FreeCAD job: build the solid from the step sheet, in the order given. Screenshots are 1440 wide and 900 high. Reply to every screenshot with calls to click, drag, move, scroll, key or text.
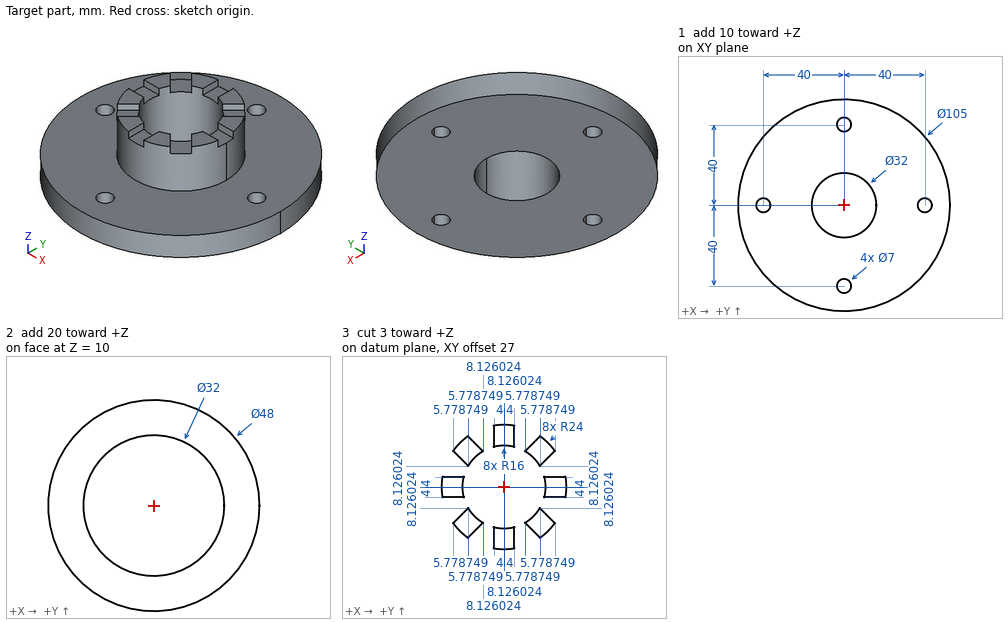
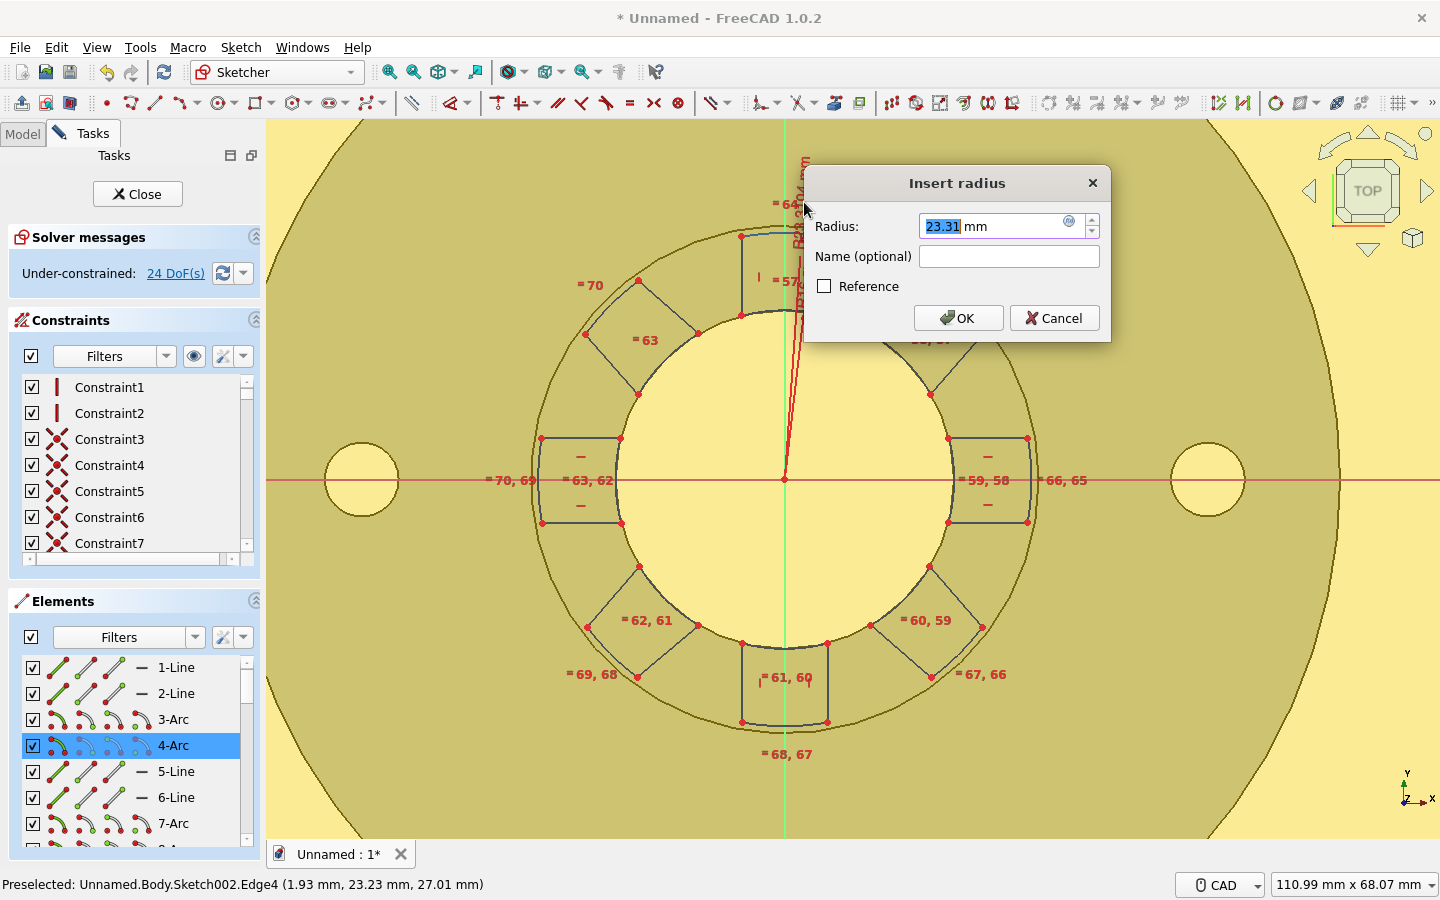
text(24)
key(Return)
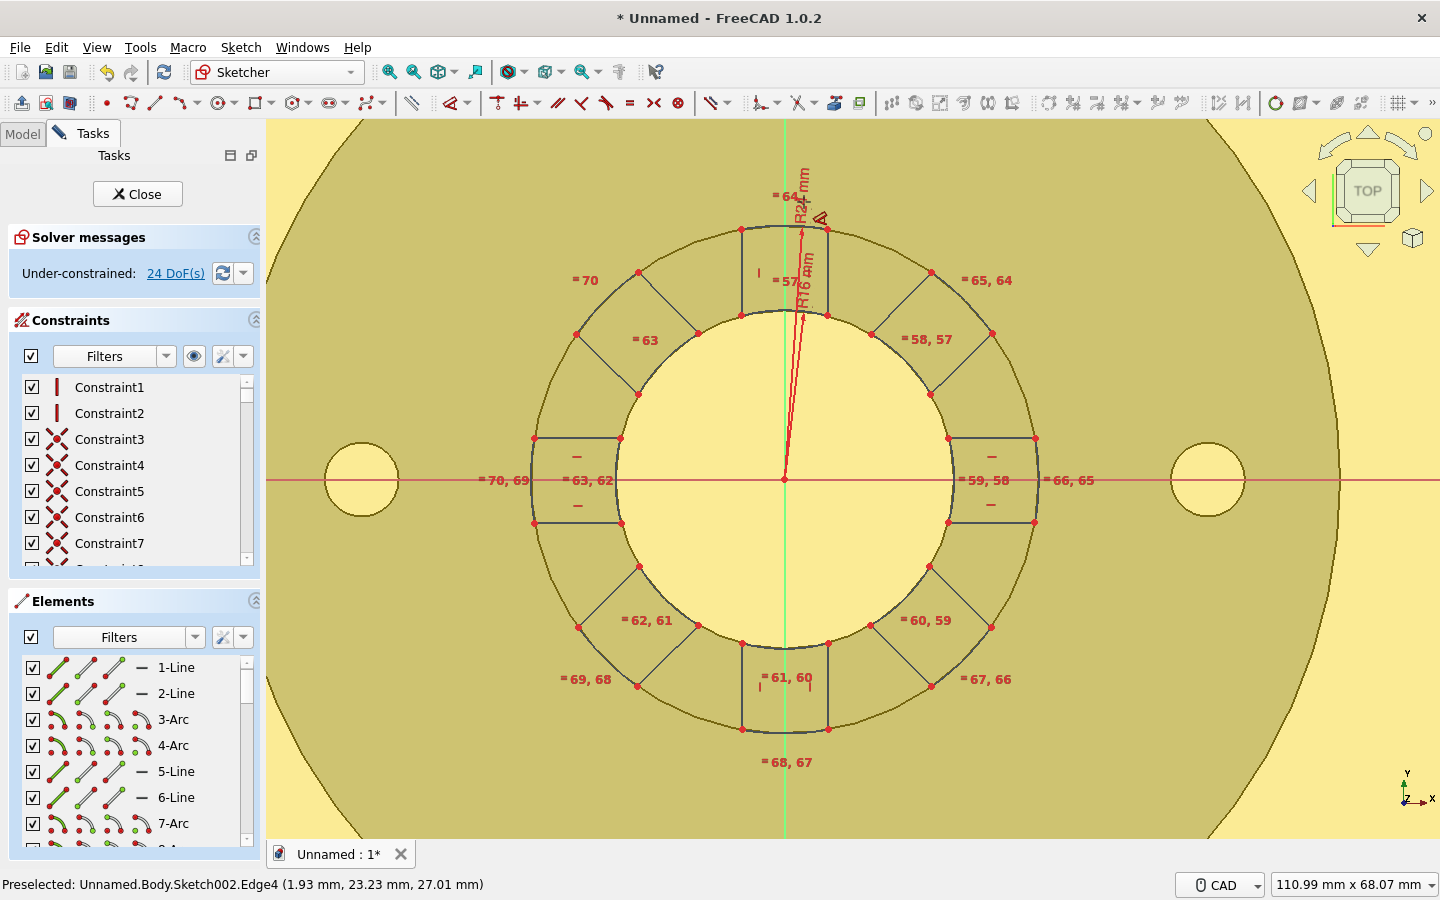
click(742, 229)
click(763, 514)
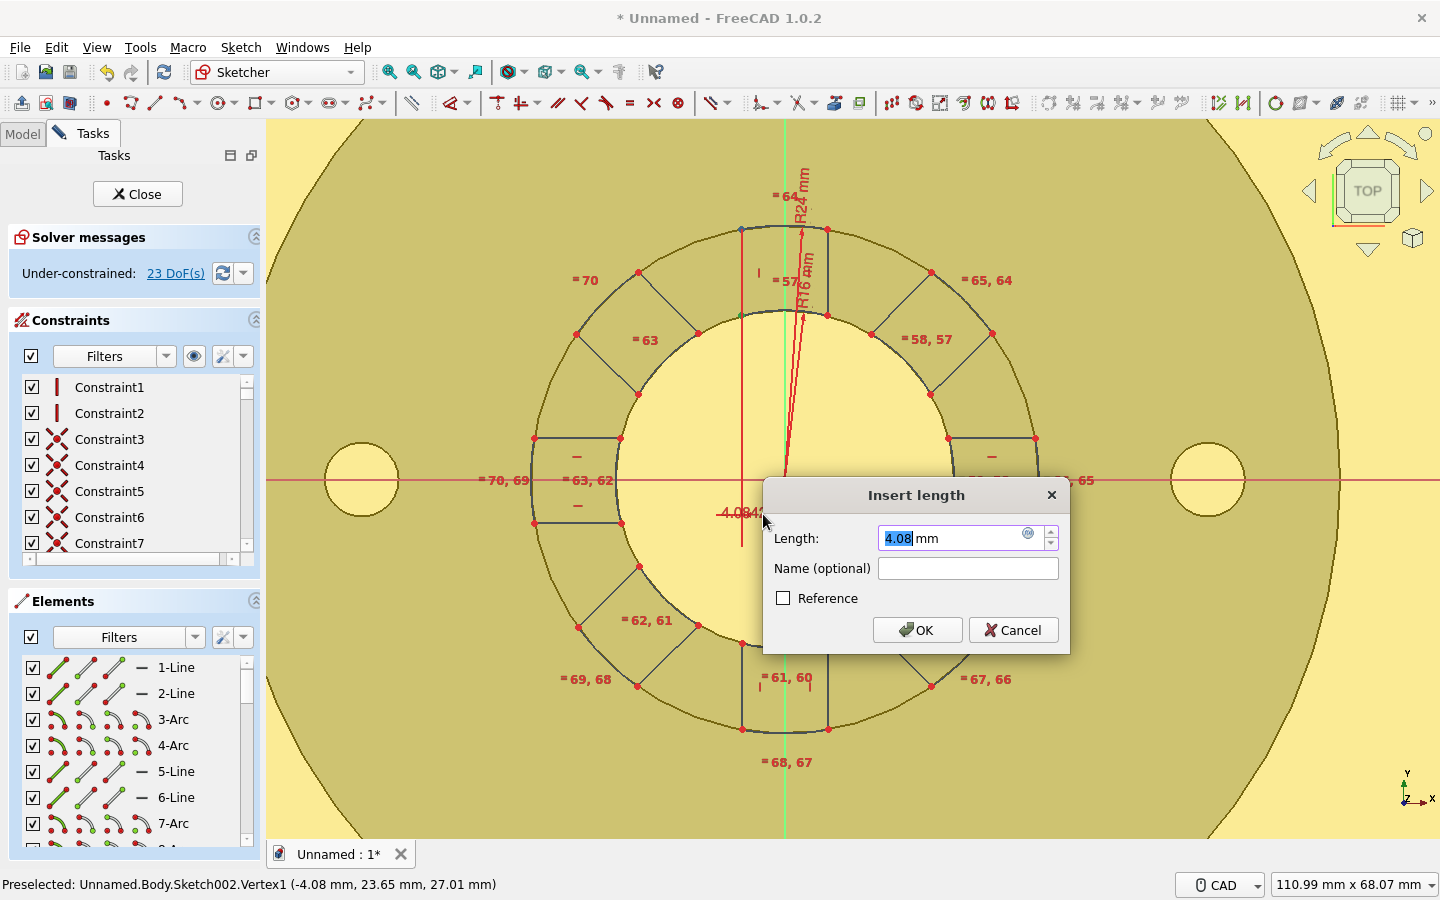
text(4)
key(Return)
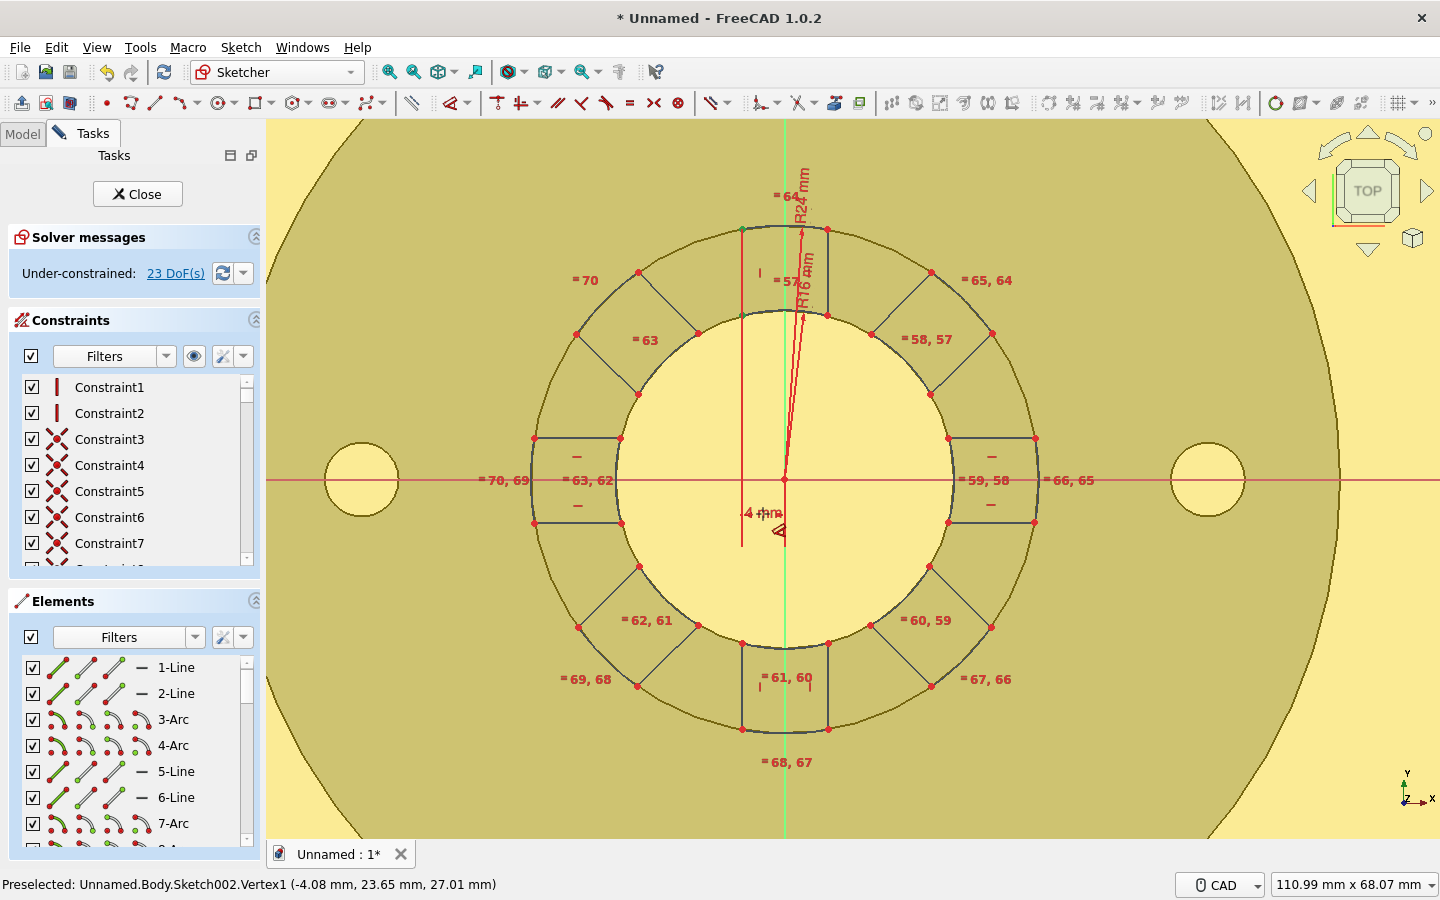
click(828, 316)
click(806, 258)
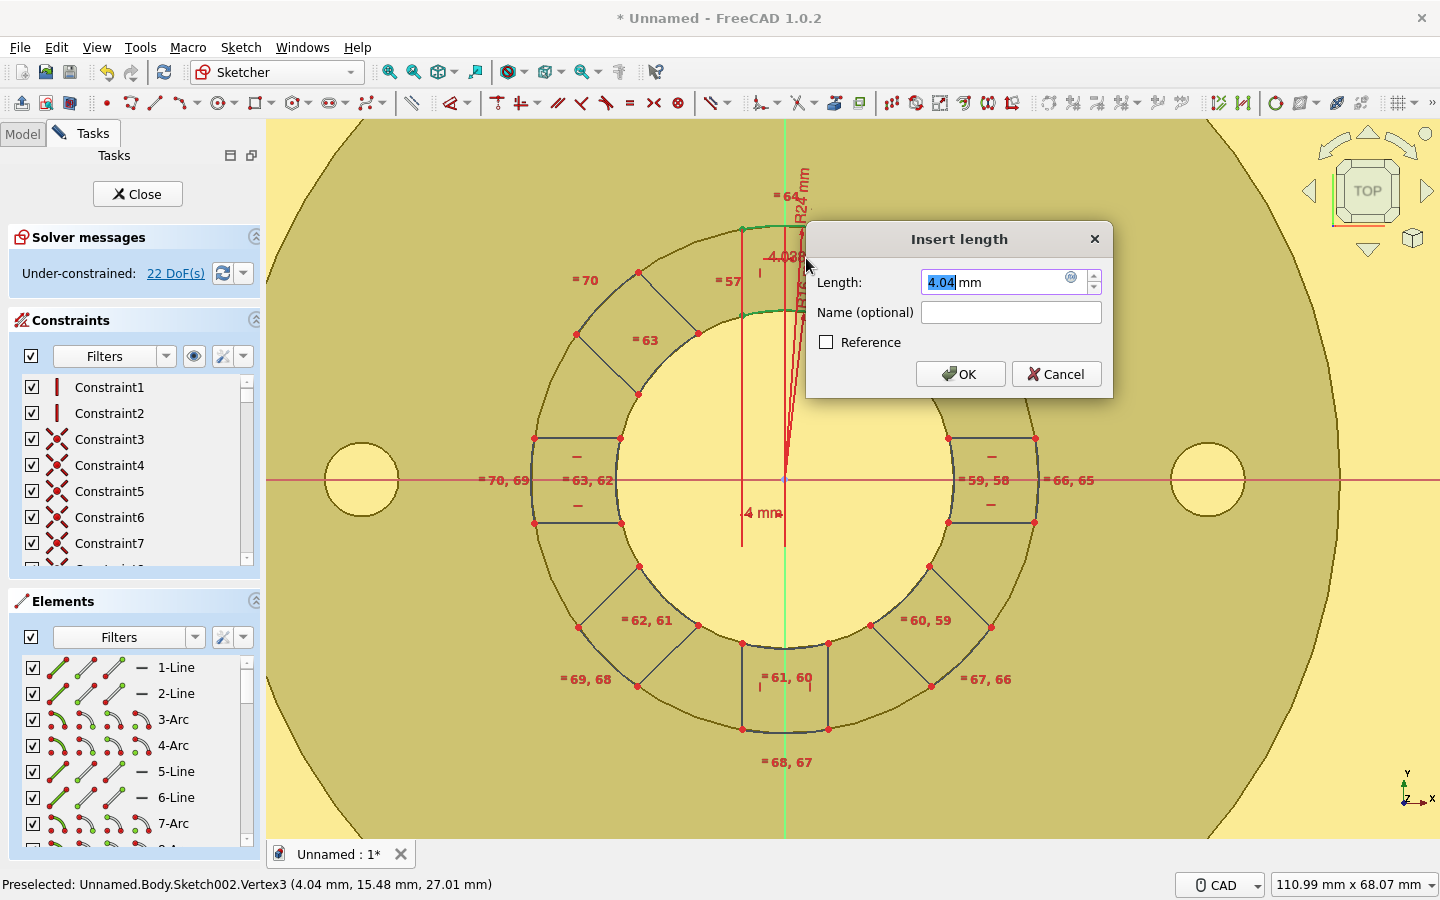
text(4)
key(Return)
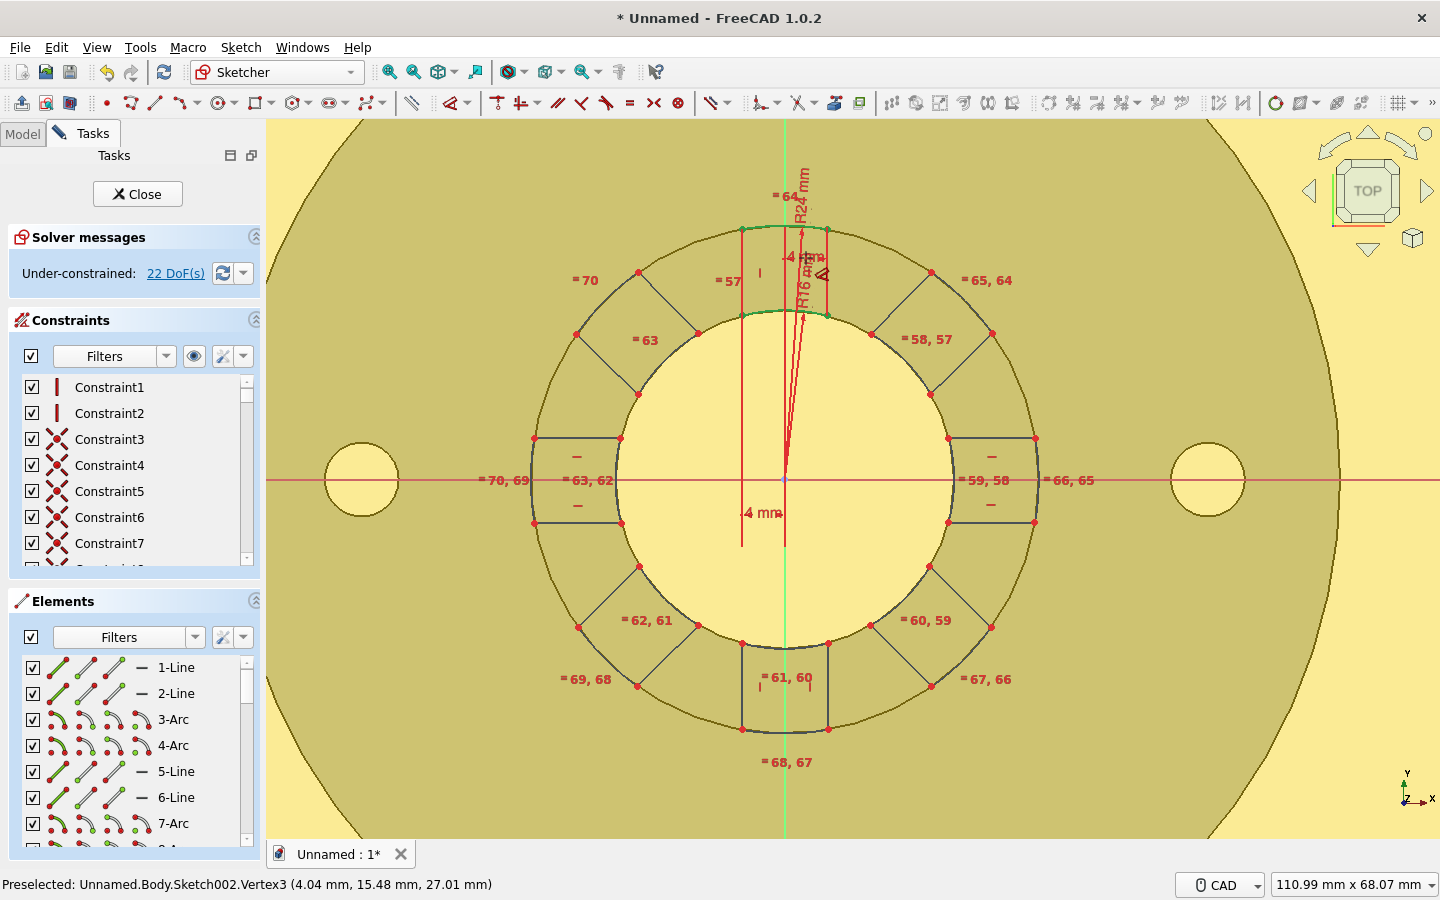
click(1035, 438)
click(1069, 459)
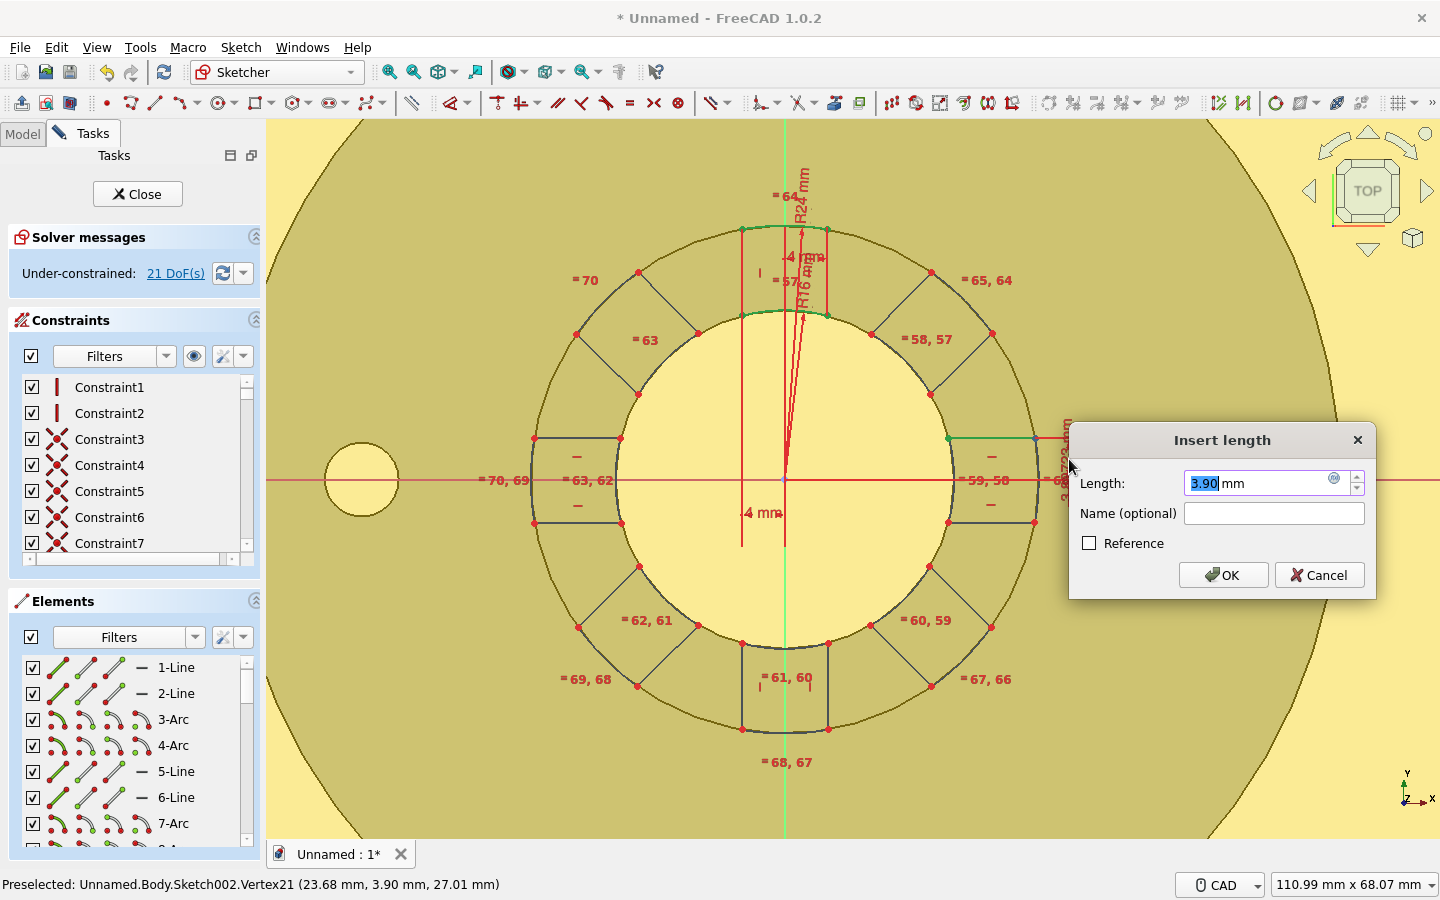
text(4)
key(Return)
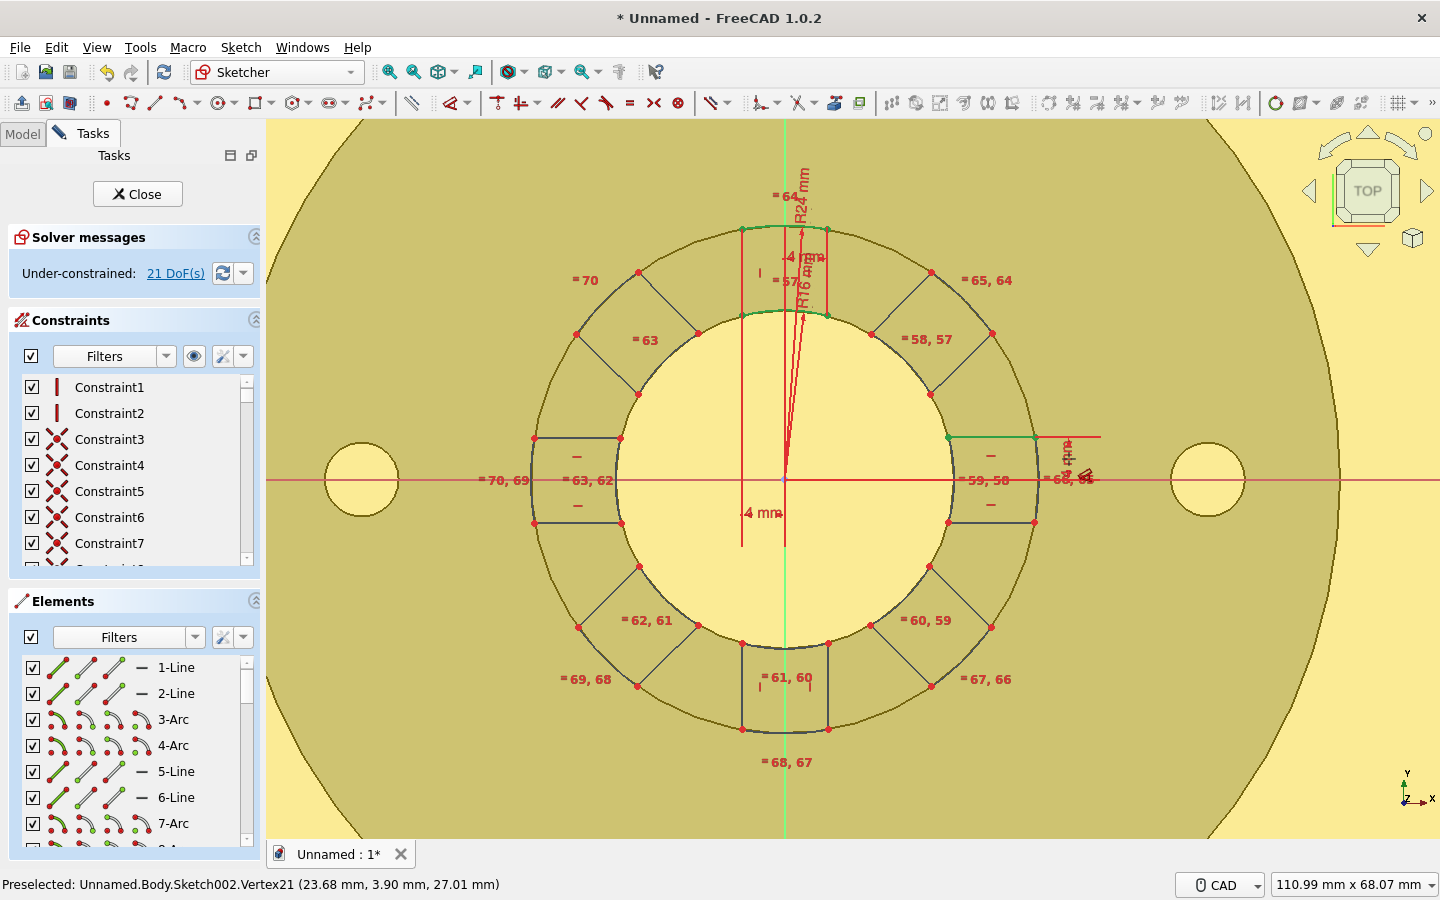
click(948, 523)
click(982, 501)